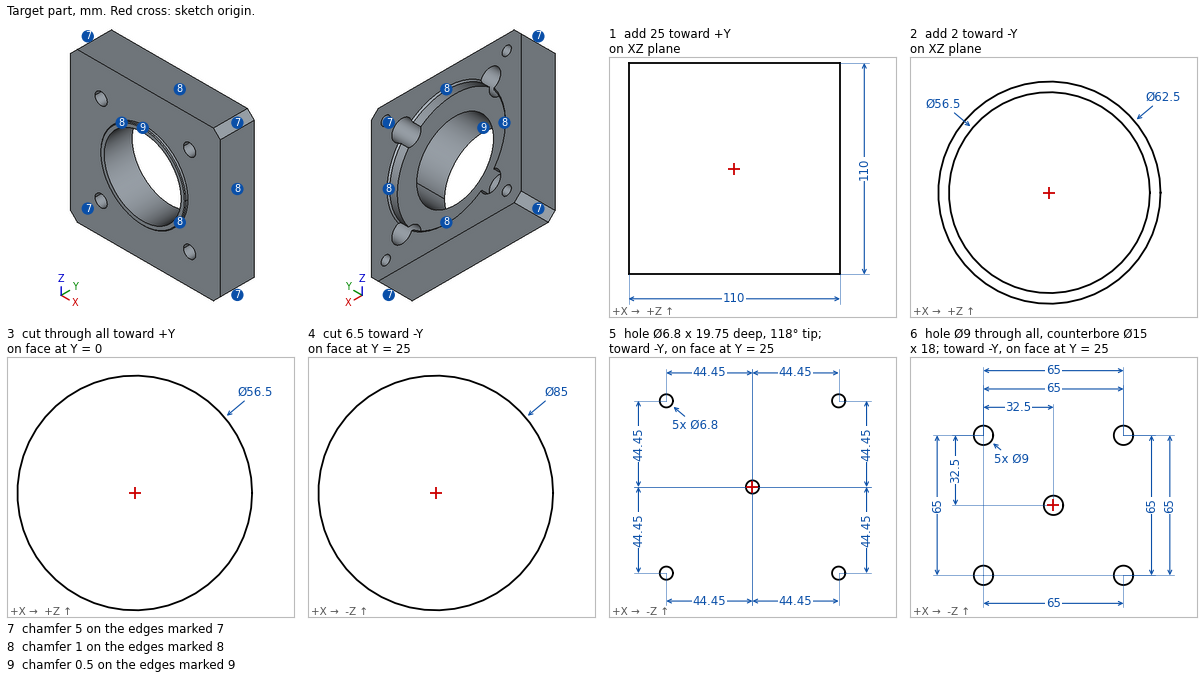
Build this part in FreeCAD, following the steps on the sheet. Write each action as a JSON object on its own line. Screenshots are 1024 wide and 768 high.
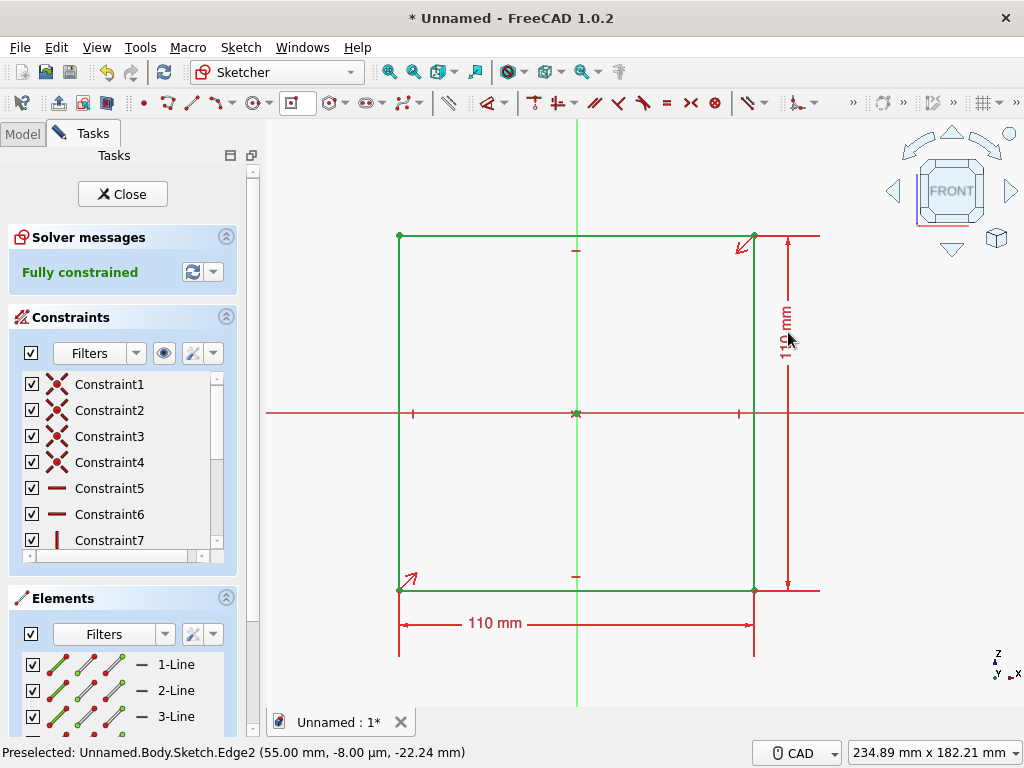
{"action": "left_click", "coordinate": [123, 194]}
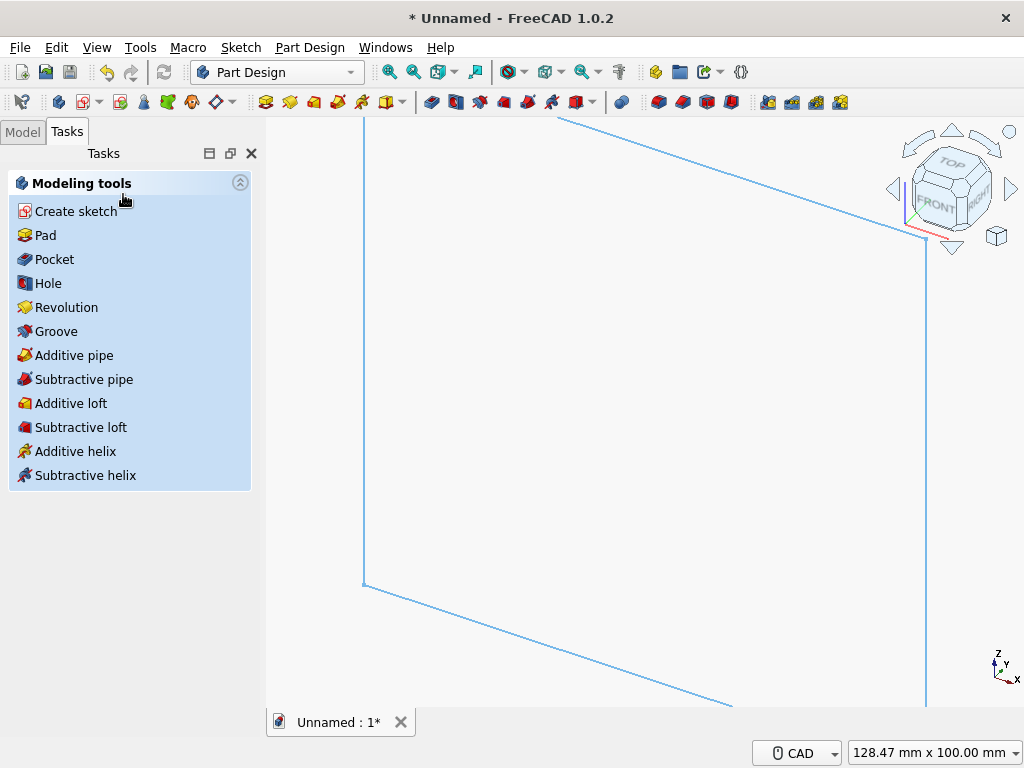
{"action": "left_click", "coordinate": [266, 102]}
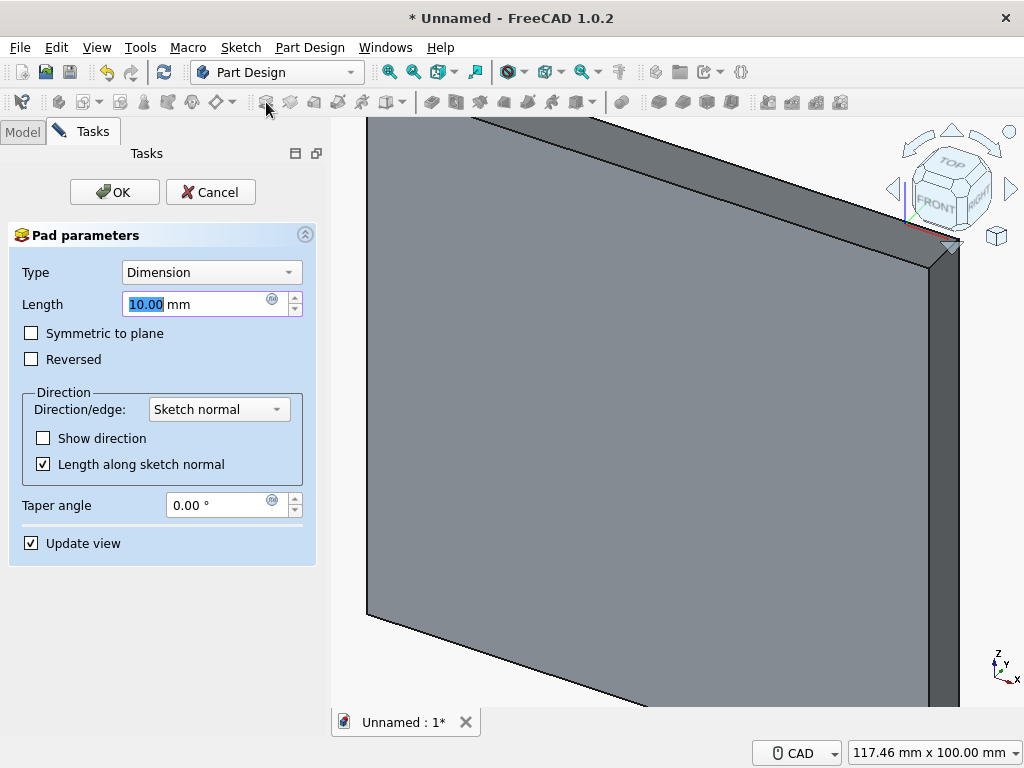
{"action": "type", "text": "25"}
{"action": "key", "text": "Tab"}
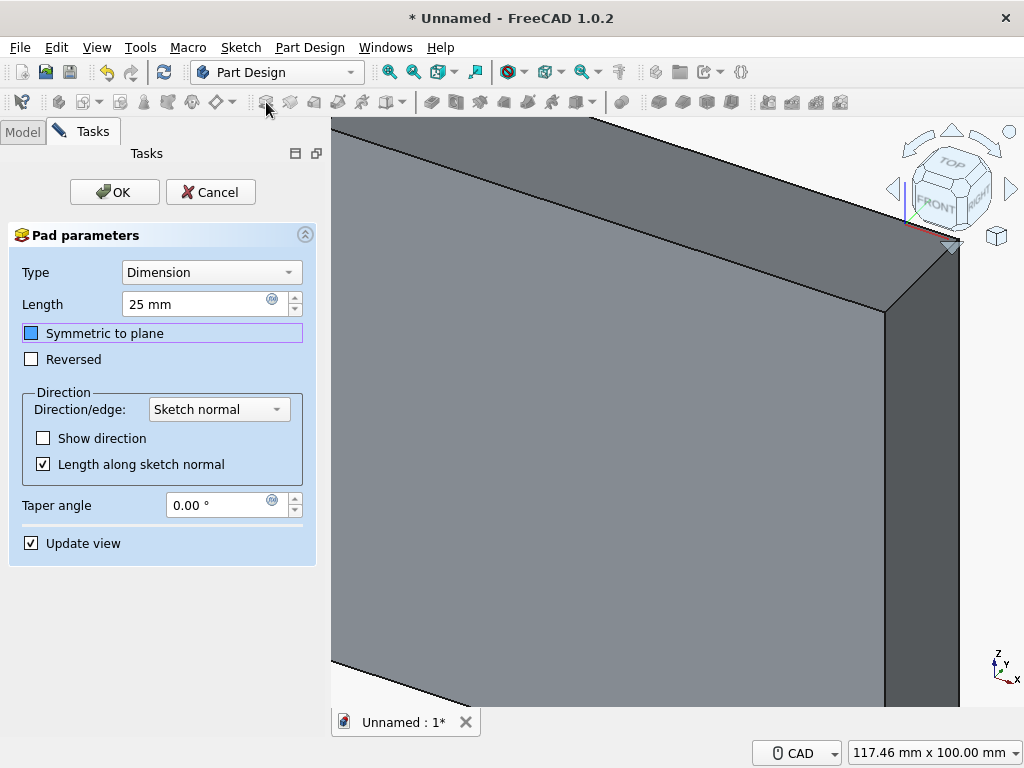
{"action": "left_click", "coordinate": [30, 359]}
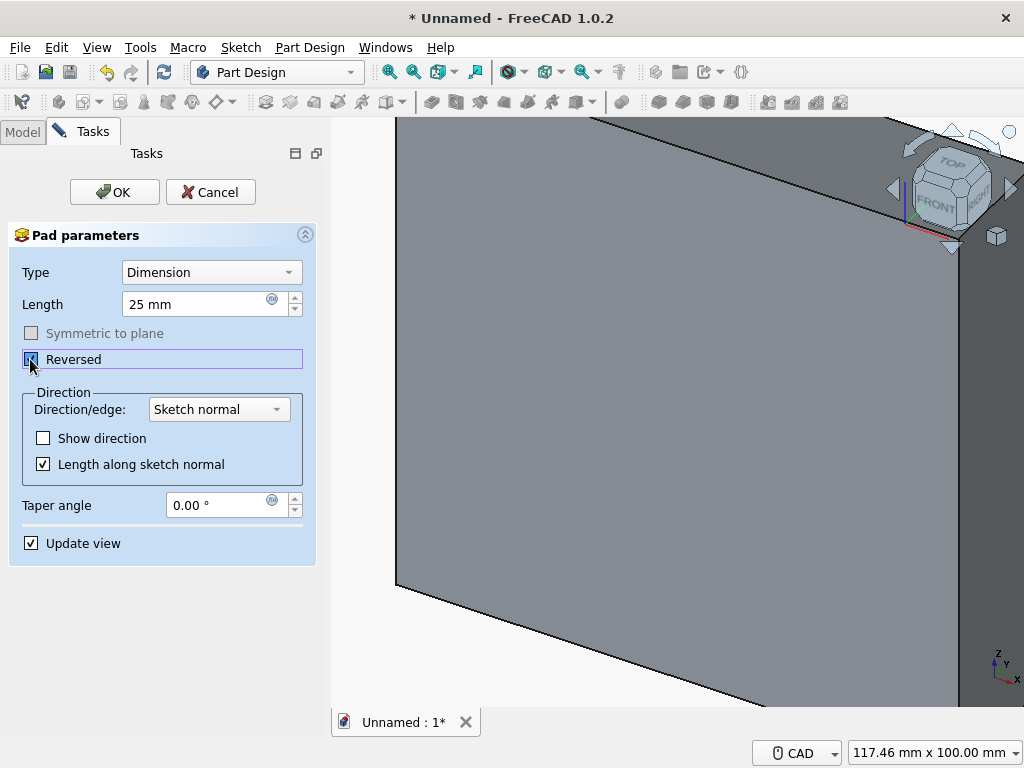
{"action": "left_click", "coordinate": [115, 192]}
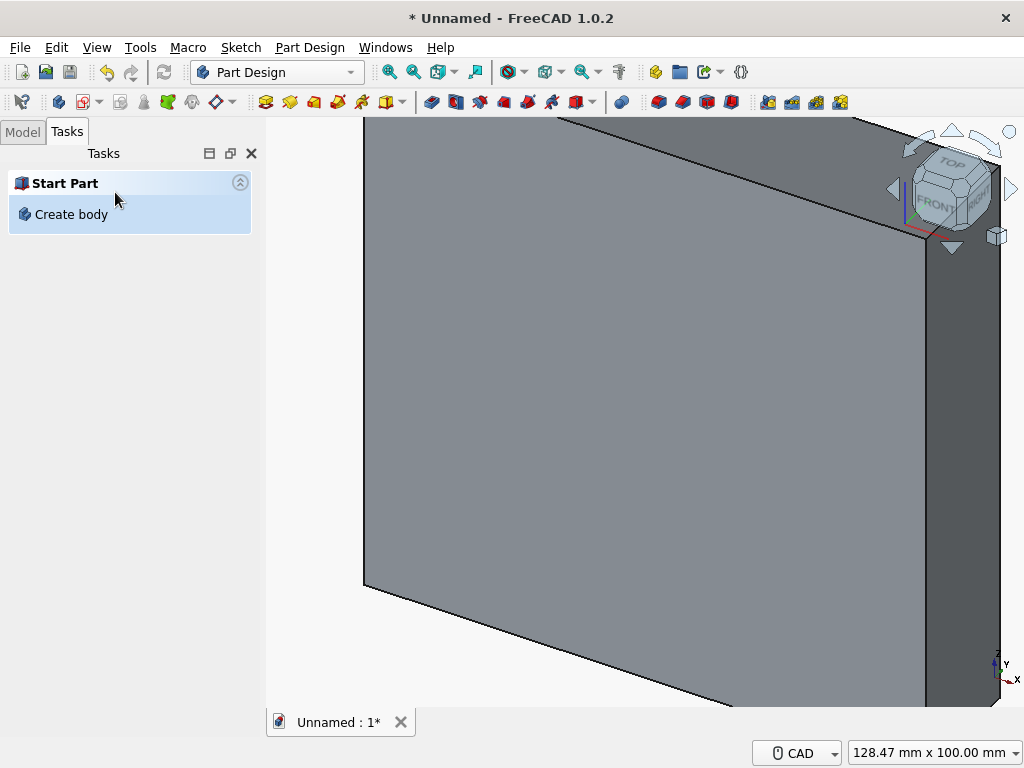
{"action": "left_click", "coordinate": [390, 72]}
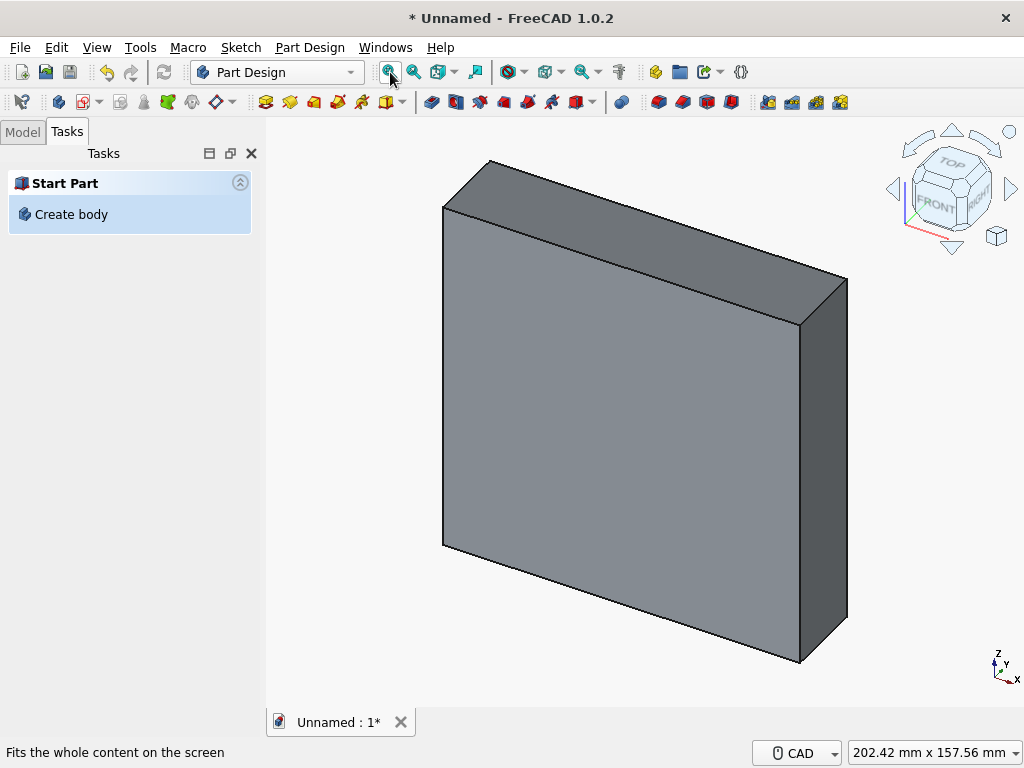
{"action": "left_click", "coordinate": [84, 102]}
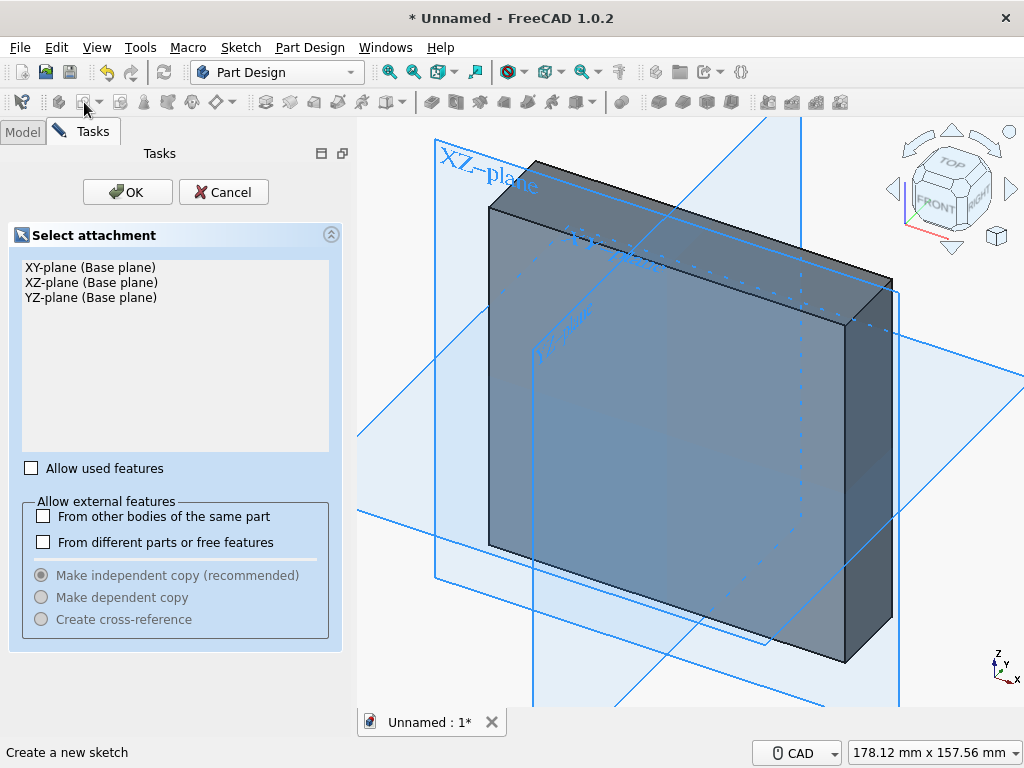
{"action": "left_click", "coordinate": [82, 282]}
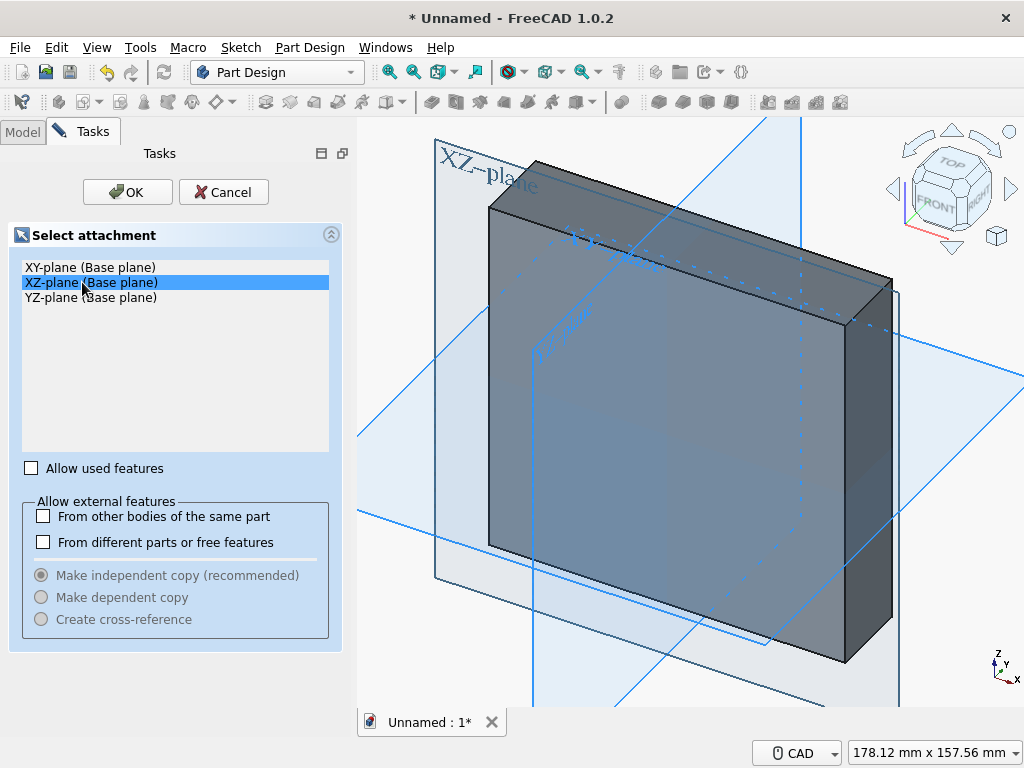
{"action": "left_click", "coordinate": [128, 192]}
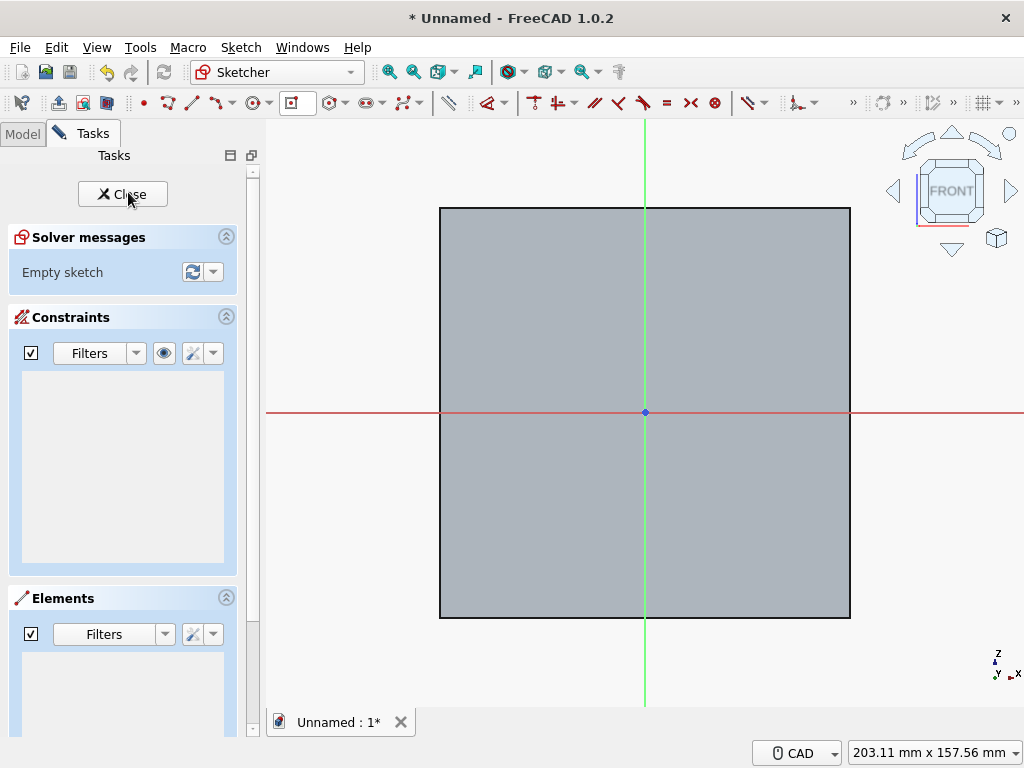
{"action": "scroll", "coordinate": [784, 413], "scroll_direction": "up", "scroll_amount": 2}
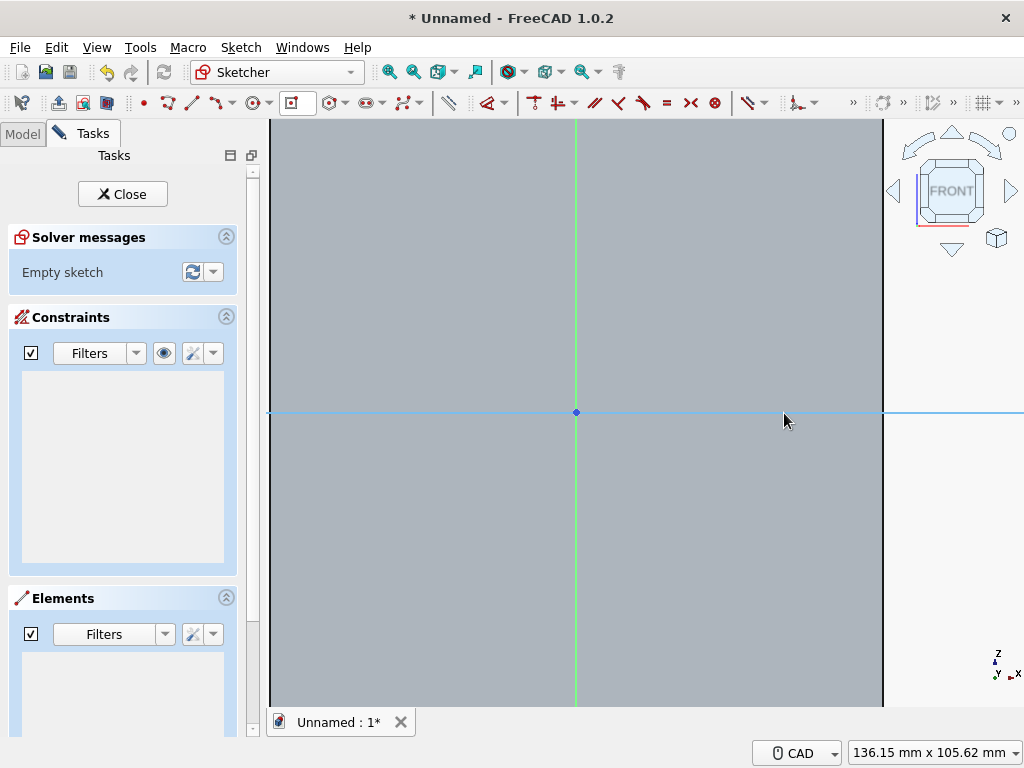
{"action": "left_click", "coordinate": [254, 104]}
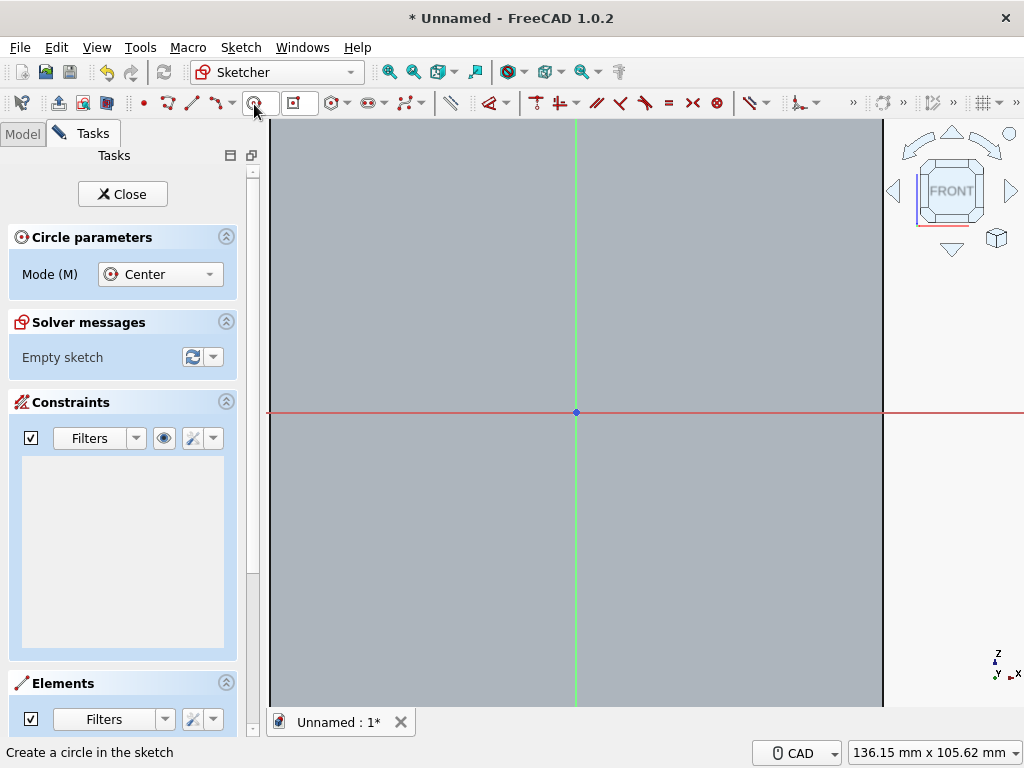
{"action": "left_click", "coordinate": [576, 413]}
{"action": "left_click", "coordinate": [699, 290]}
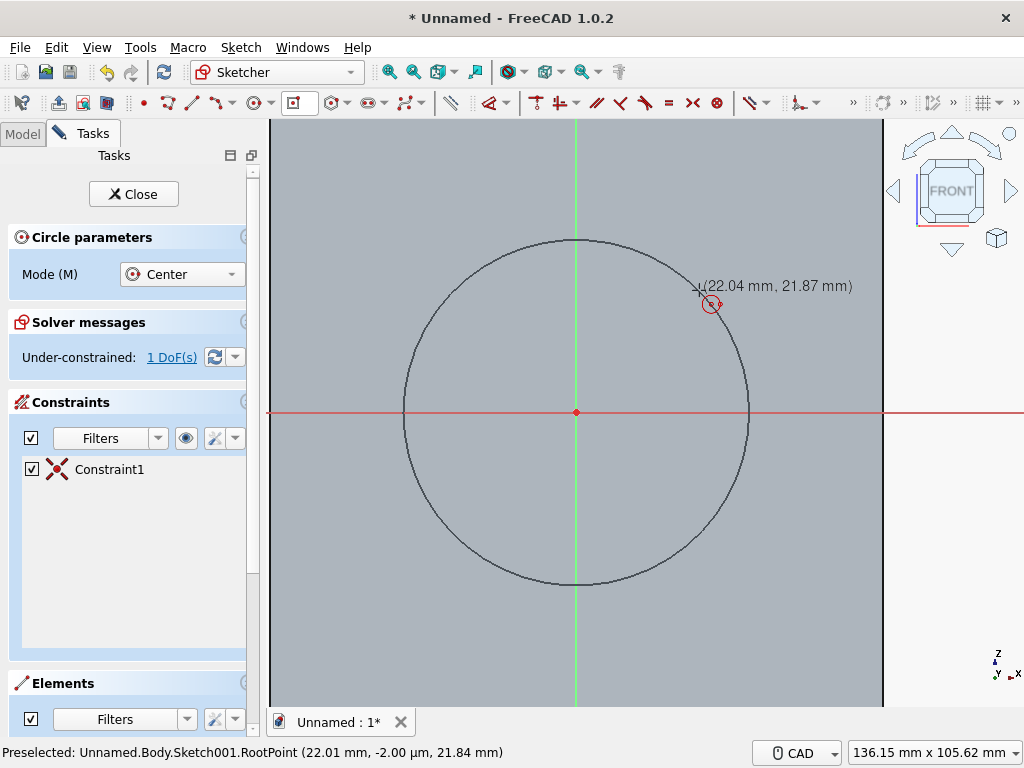
{"action": "left_click", "coordinate": [576, 413]}
{"action": "left_click", "coordinate": [688, 302]}
{"action": "key", "text": "Escape"}